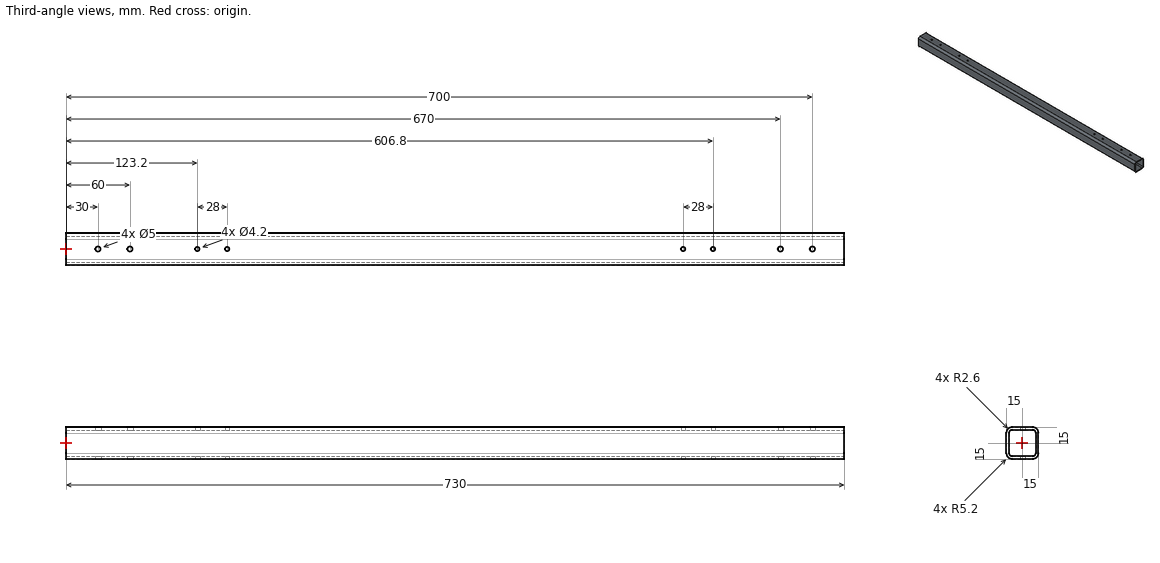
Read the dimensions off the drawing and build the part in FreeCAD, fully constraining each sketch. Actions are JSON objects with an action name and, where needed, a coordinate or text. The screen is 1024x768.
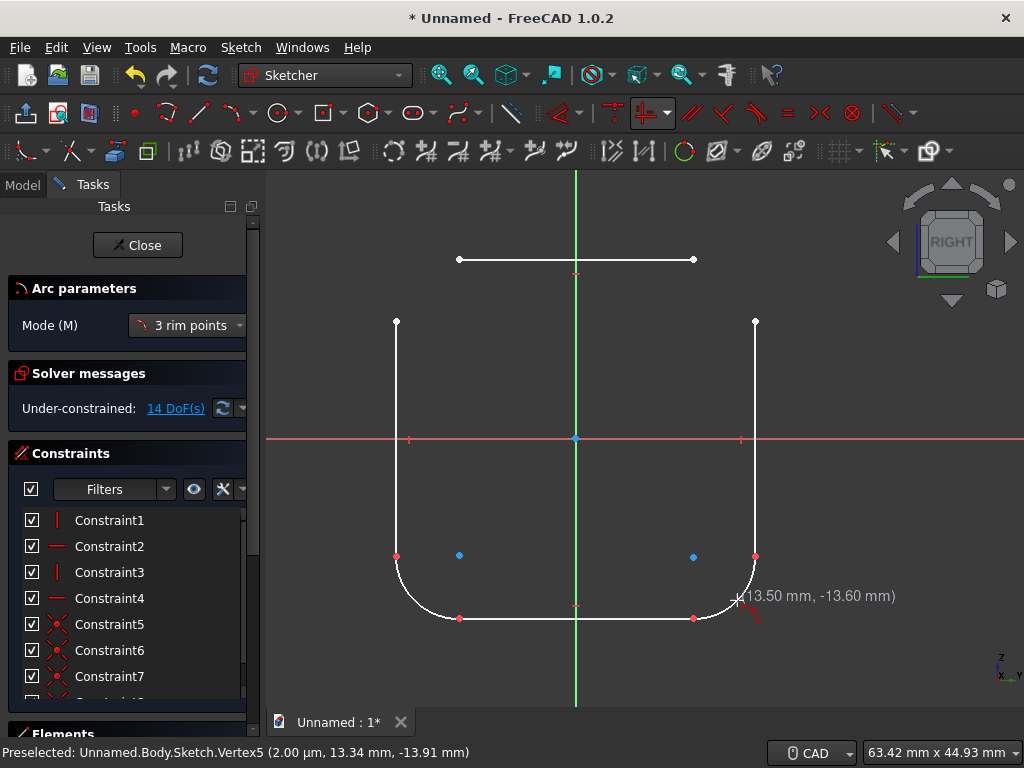
{"action": "left_click", "coordinate": [755, 322]}
{"action": "left_click", "coordinate": [693, 260]}
{"action": "left_click", "coordinate": [737, 277]}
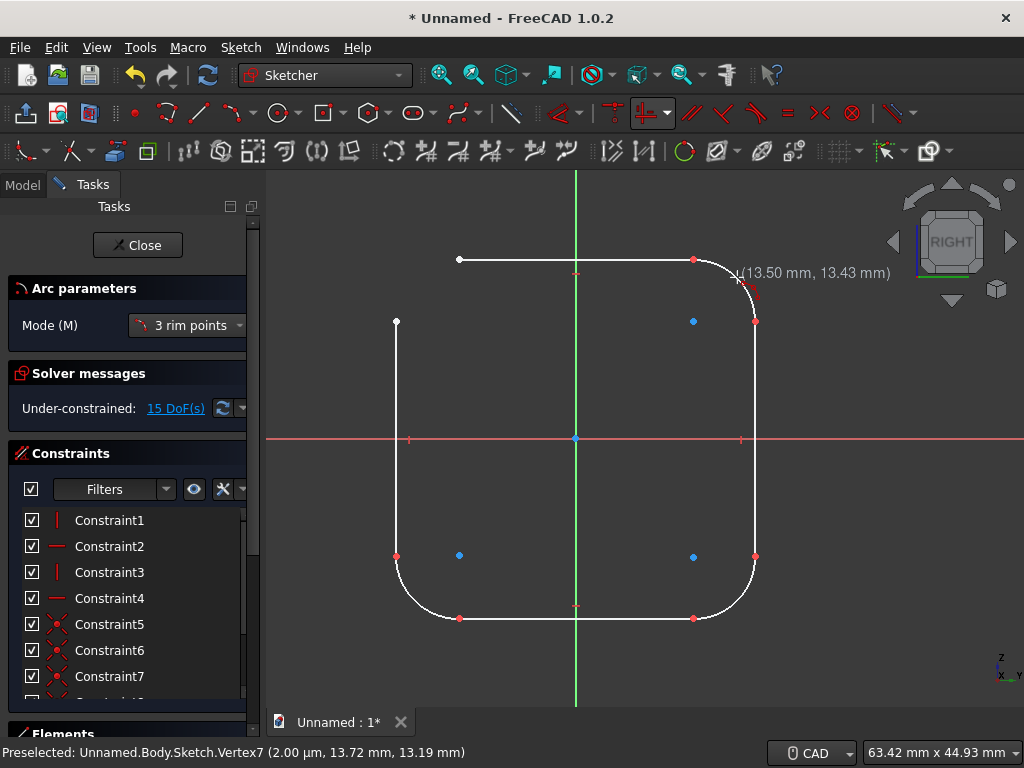
{"action": "left_click", "coordinate": [459, 260]}
{"action": "left_click", "coordinate": [396, 322]}
{"action": "left_click", "coordinate": [415, 277]}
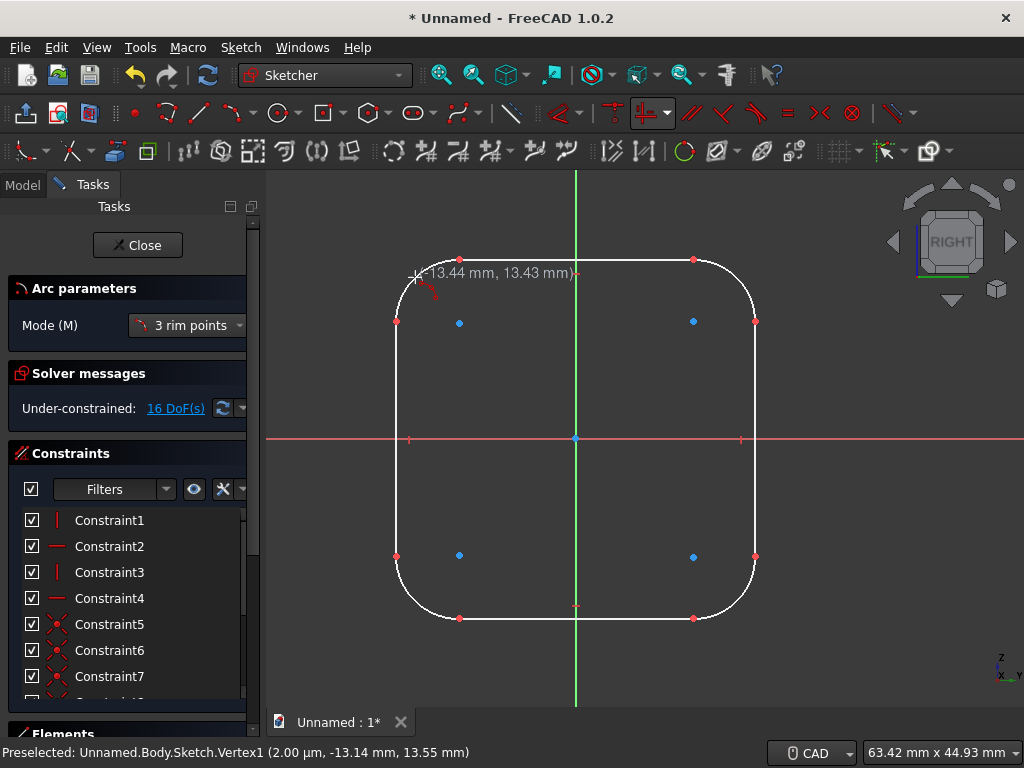
{"action": "left_click", "coordinate": [200, 114]}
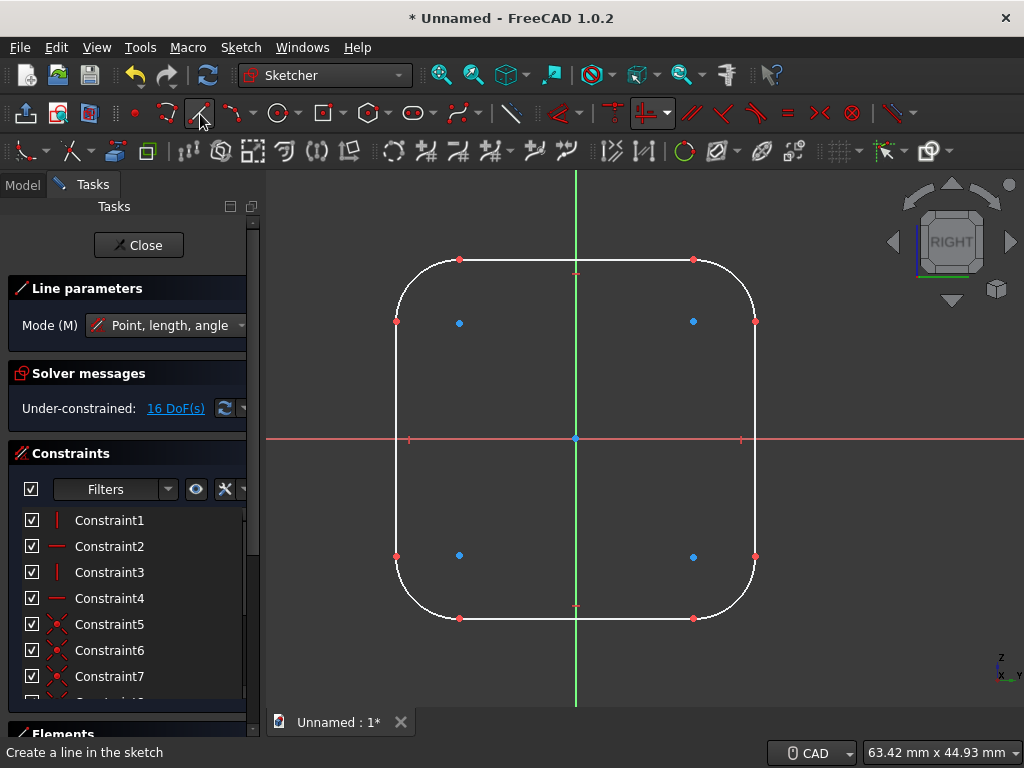
{"action": "left_click", "coordinate": [427, 556]}
{"action": "left_click", "coordinate": [427, 321]}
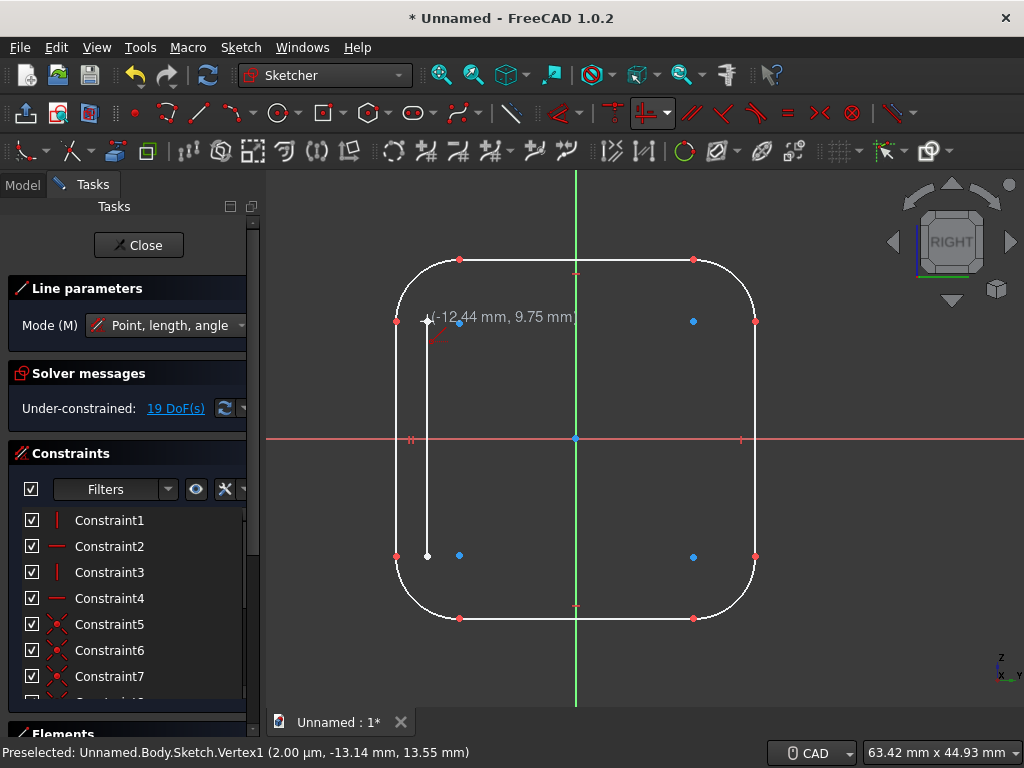
{"action": "left_click", "coordinate": [459, 290]}
{"action": "left_click", "coordinate": [693, 290]}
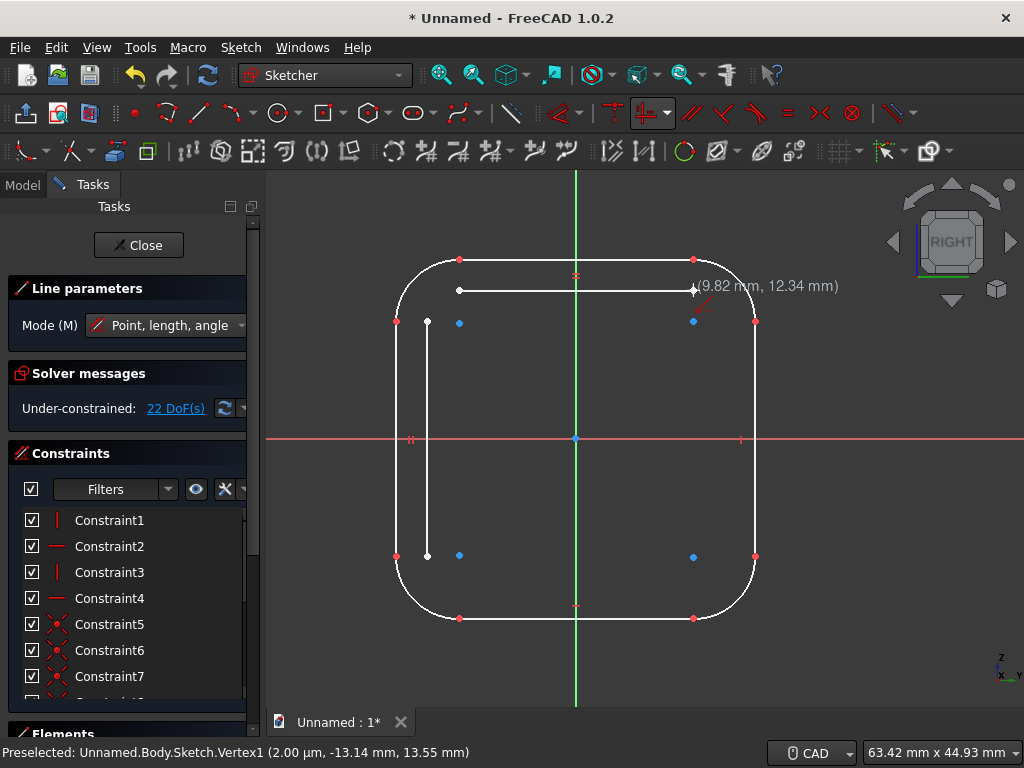
{"action": "left_click", "coordinate": [724, 321]}
{"action": "left_click", "coordinate": [724, 556]}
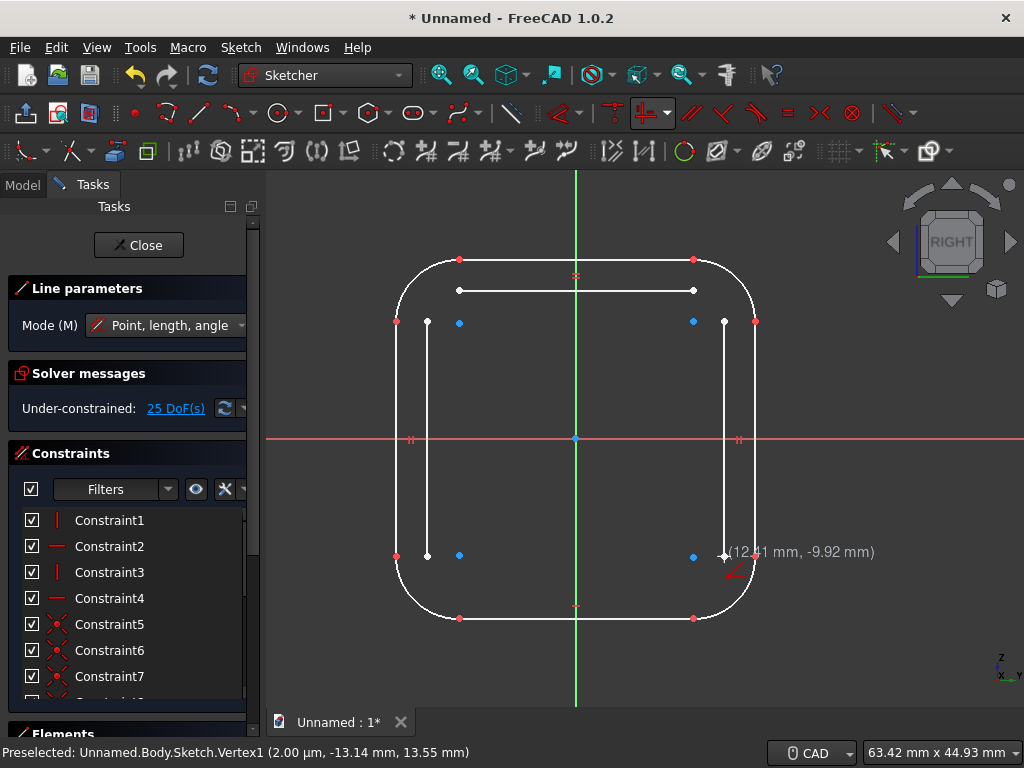
{"action": "left_click", "coordinate": [693, 587]}
{"action": "left_click", "coordinate": [459, 587]}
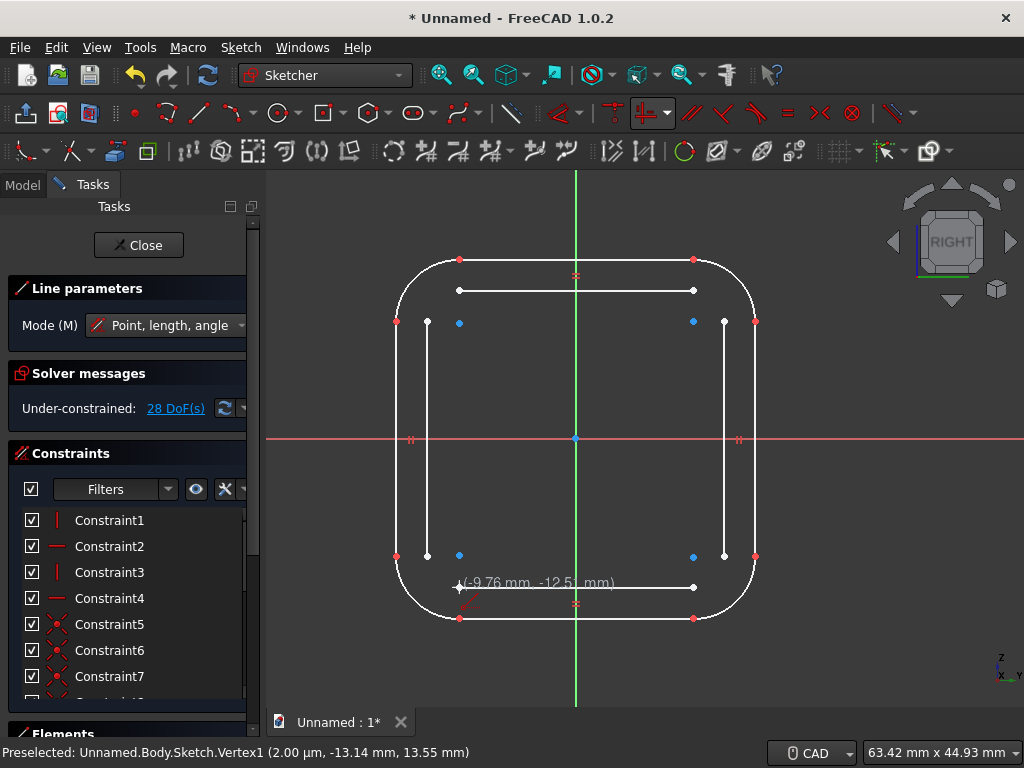
{"action": "left_click", "coordinate": [232, 114]}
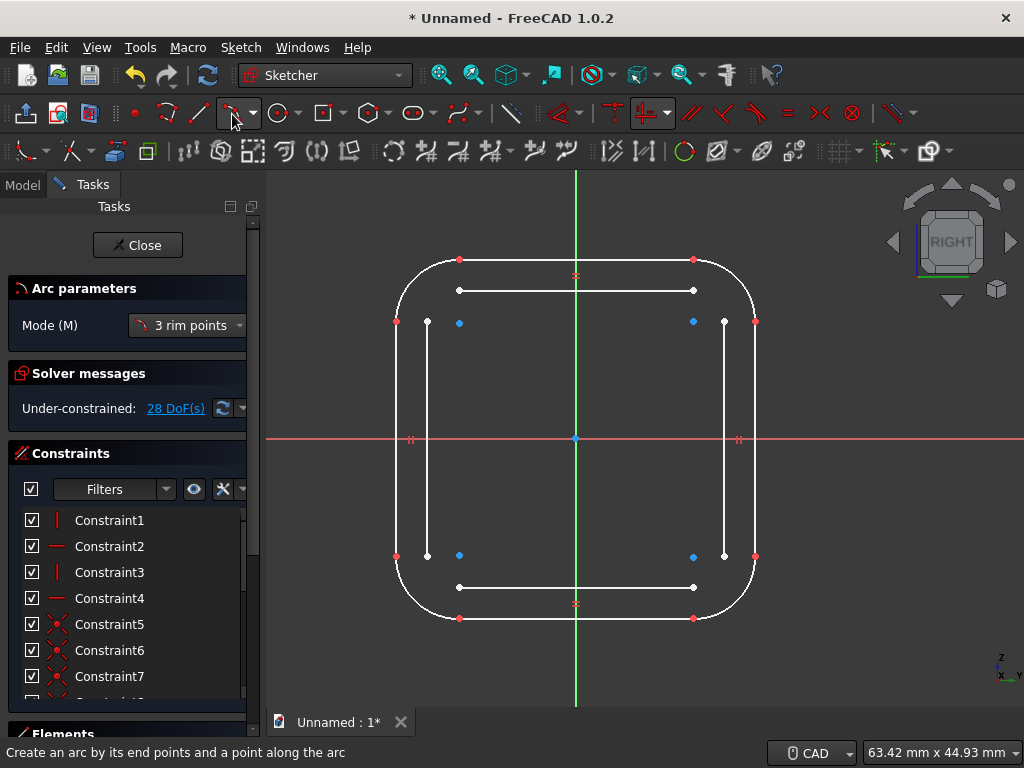
{"action": "left_click", "coordinate": [427, 322]}
{"action": "left_click", "coordinate": [459, 291]}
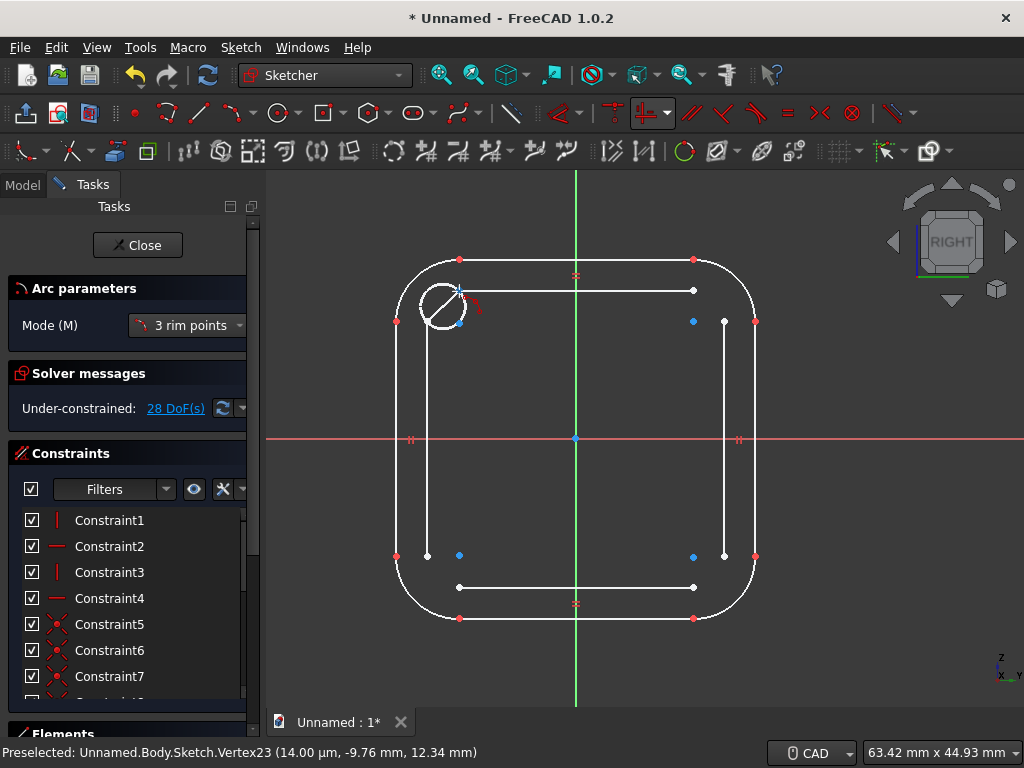
{"action": "scroll", "coordinate": [437, 299], "scroll_direction": "up", "scroll_amount": 3}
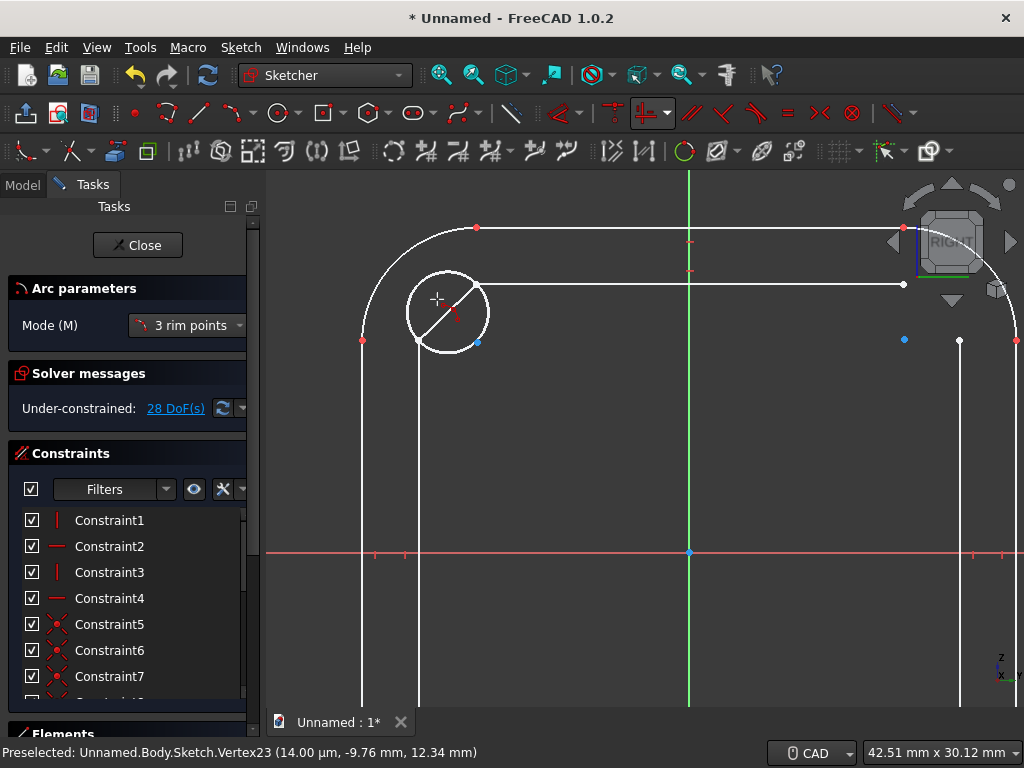
{"action": "left_click", "coordinate": [436, 300]}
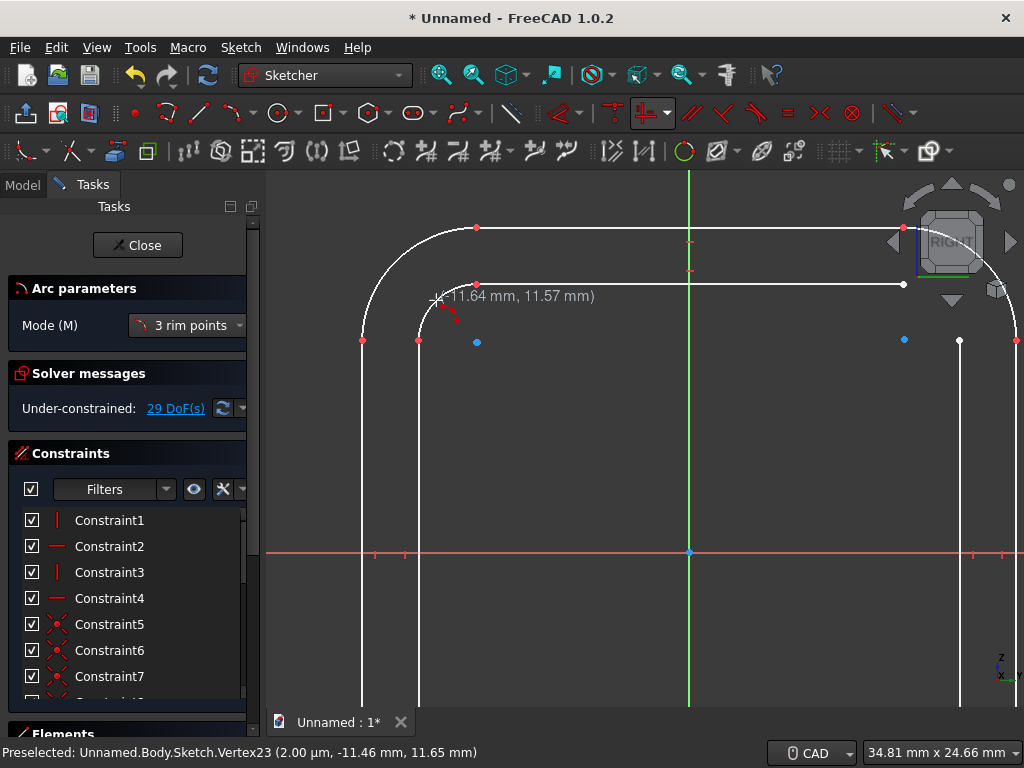
{"action": "scroll", "coordinate": [439, 299], "scroll_direction": "down", "scroll_amount": 3}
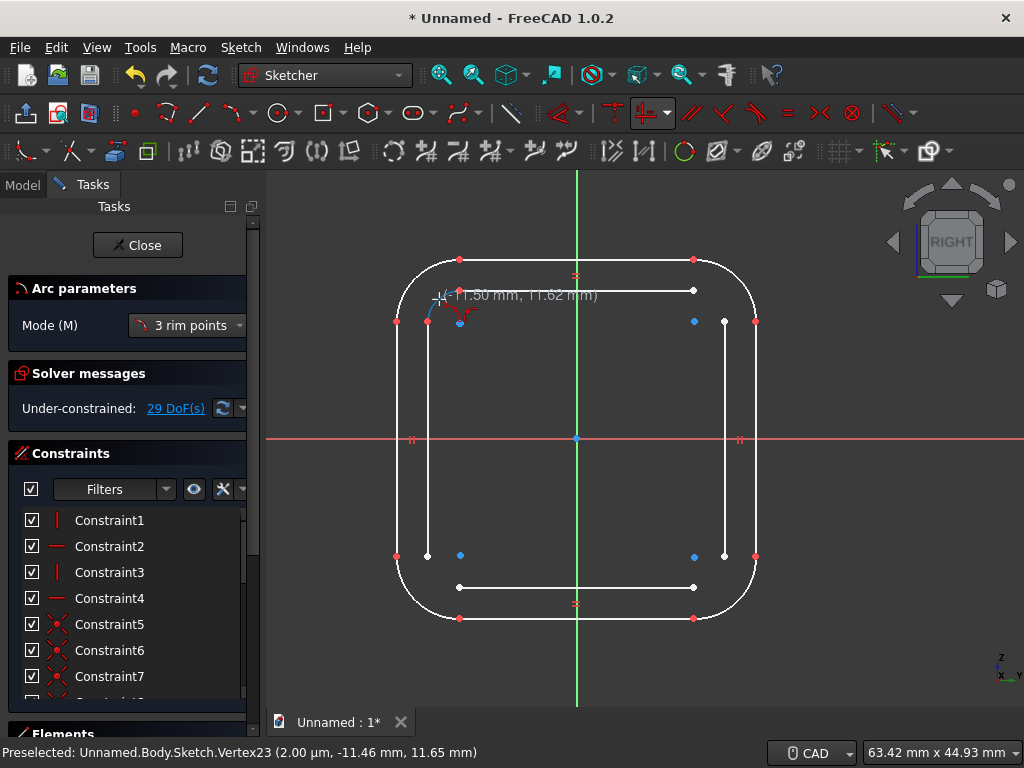
{"action": "left_click", "coordinate": [694, 291]}
{"action": "left_click", "coordinate": [725, 322]}